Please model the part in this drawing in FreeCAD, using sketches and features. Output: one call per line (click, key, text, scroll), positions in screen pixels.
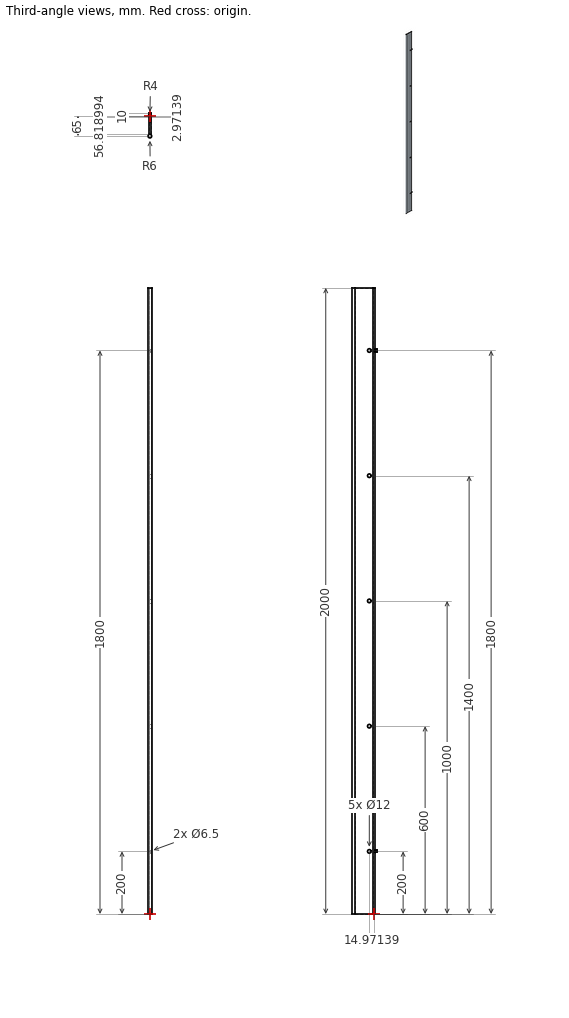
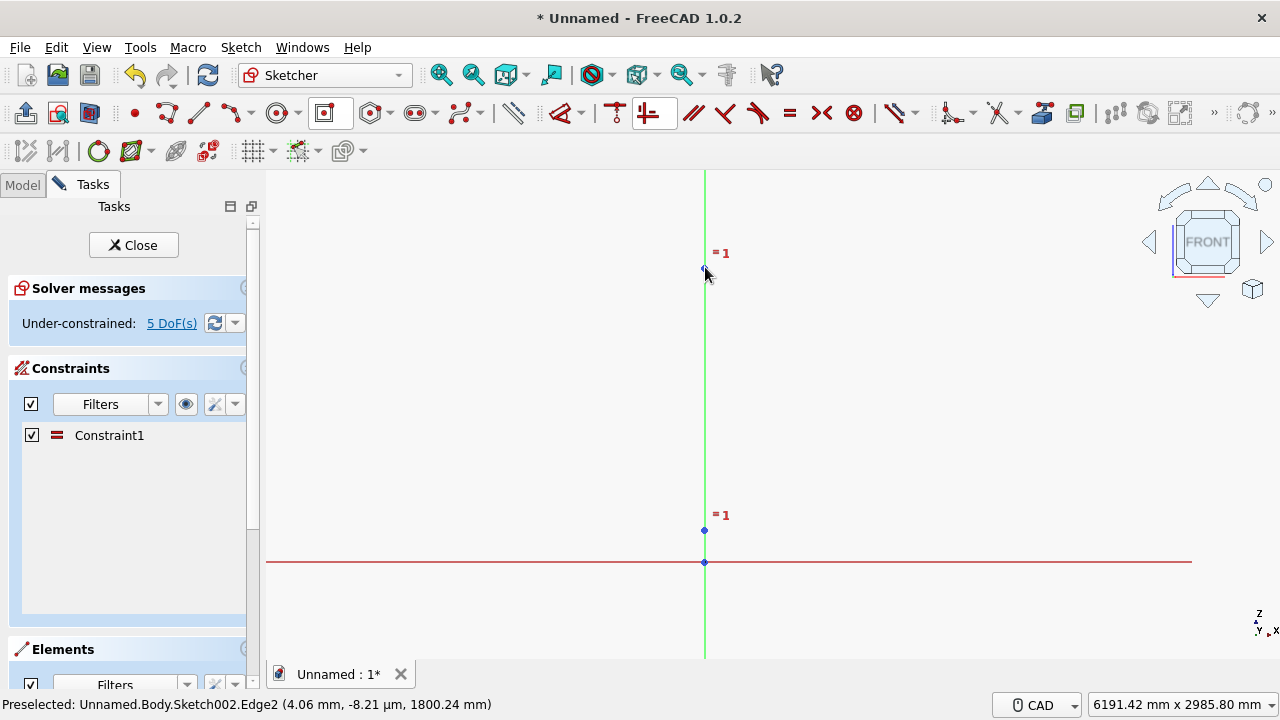
click(704, 531)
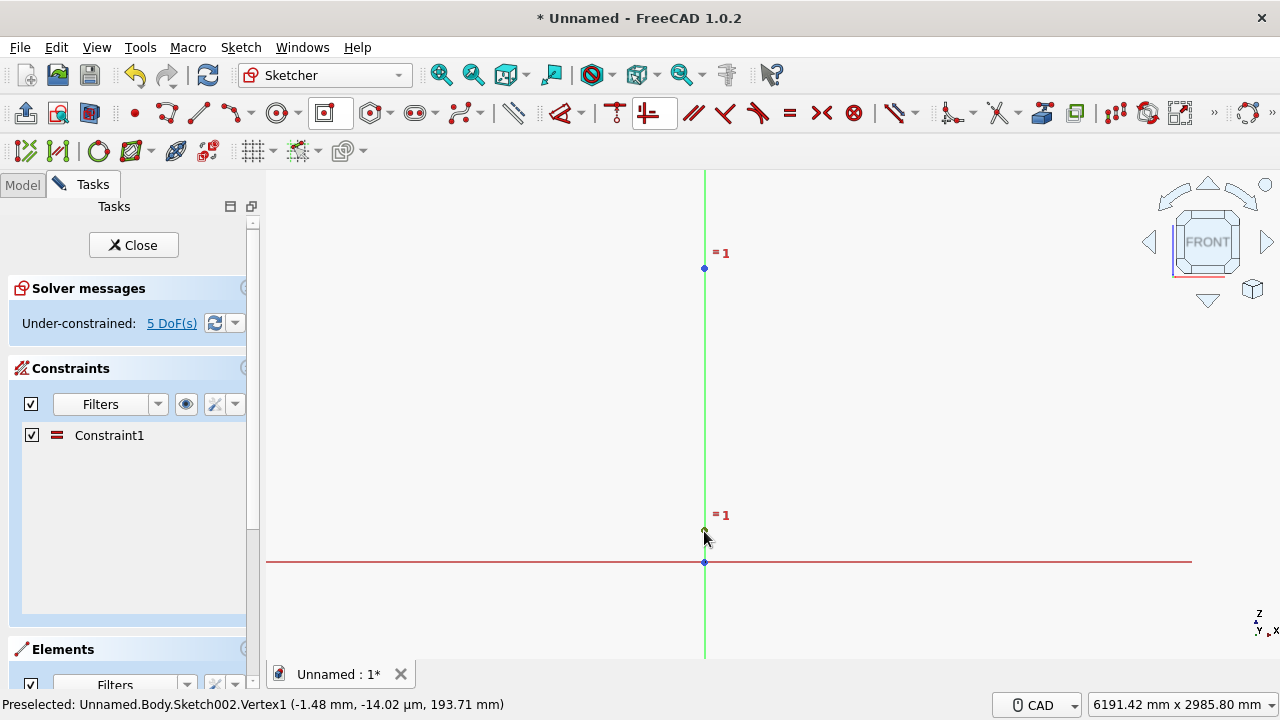
click(705, 600)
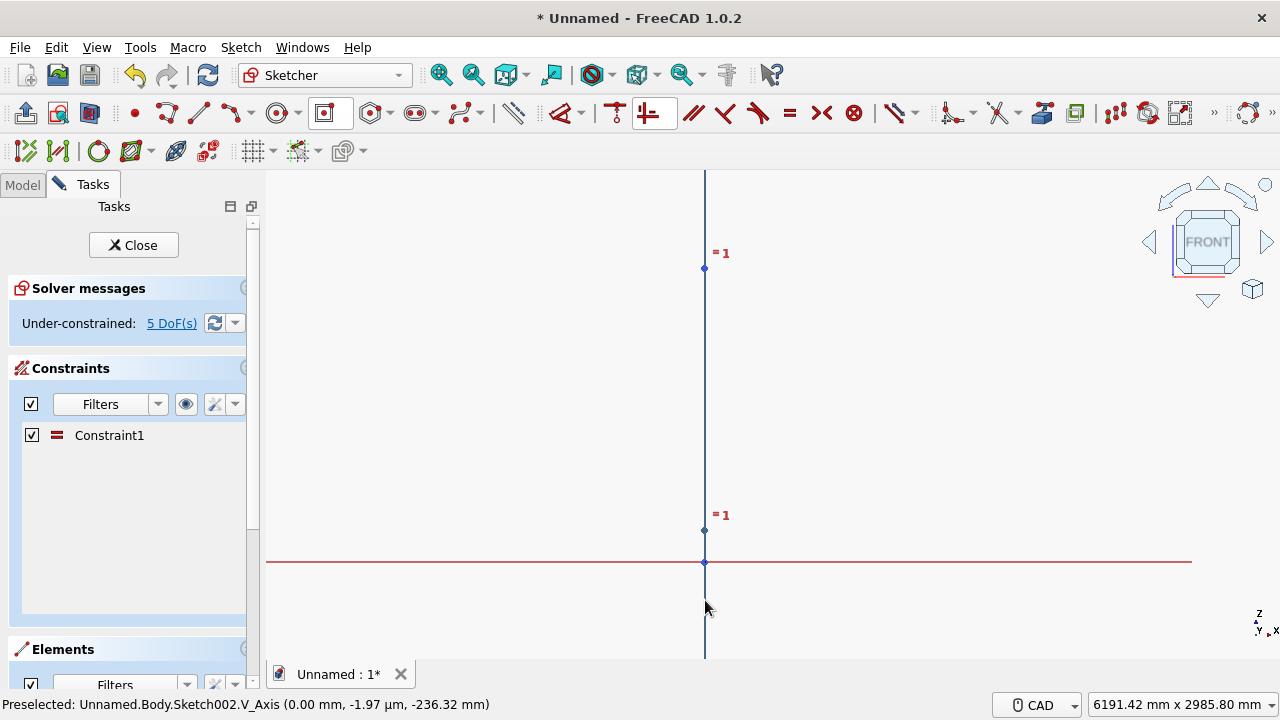
key(c)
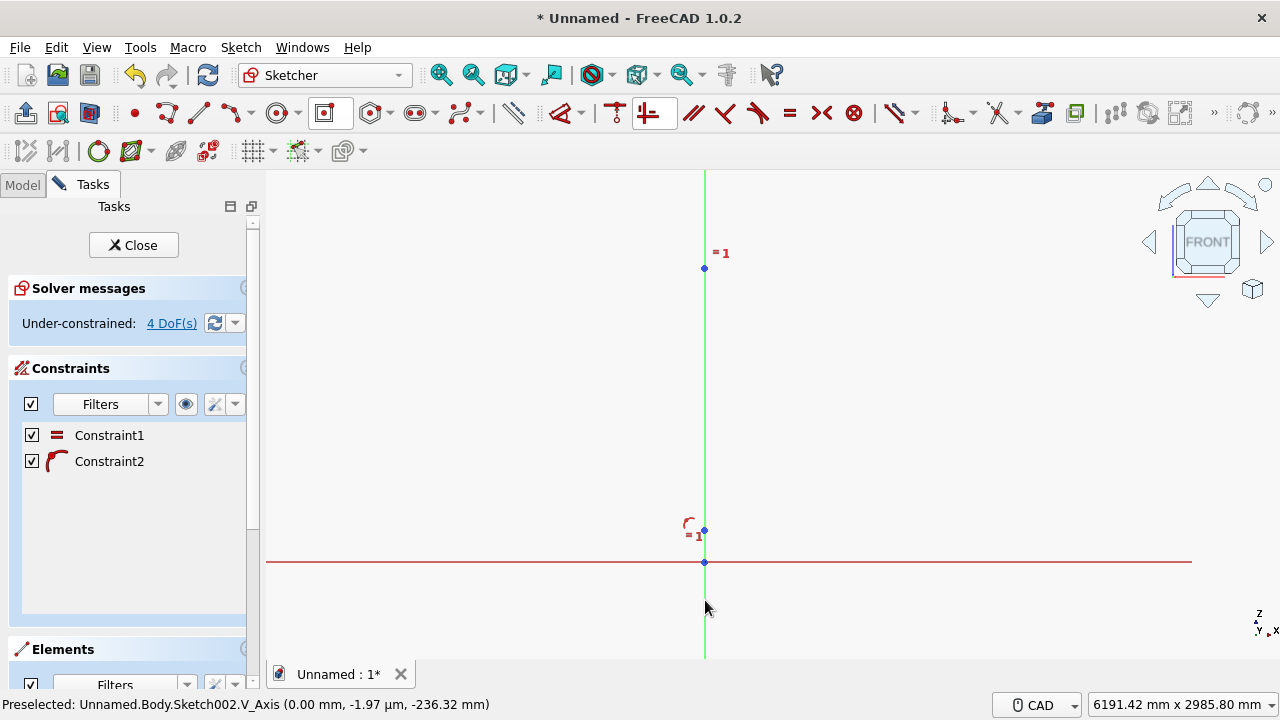
click(704, 269)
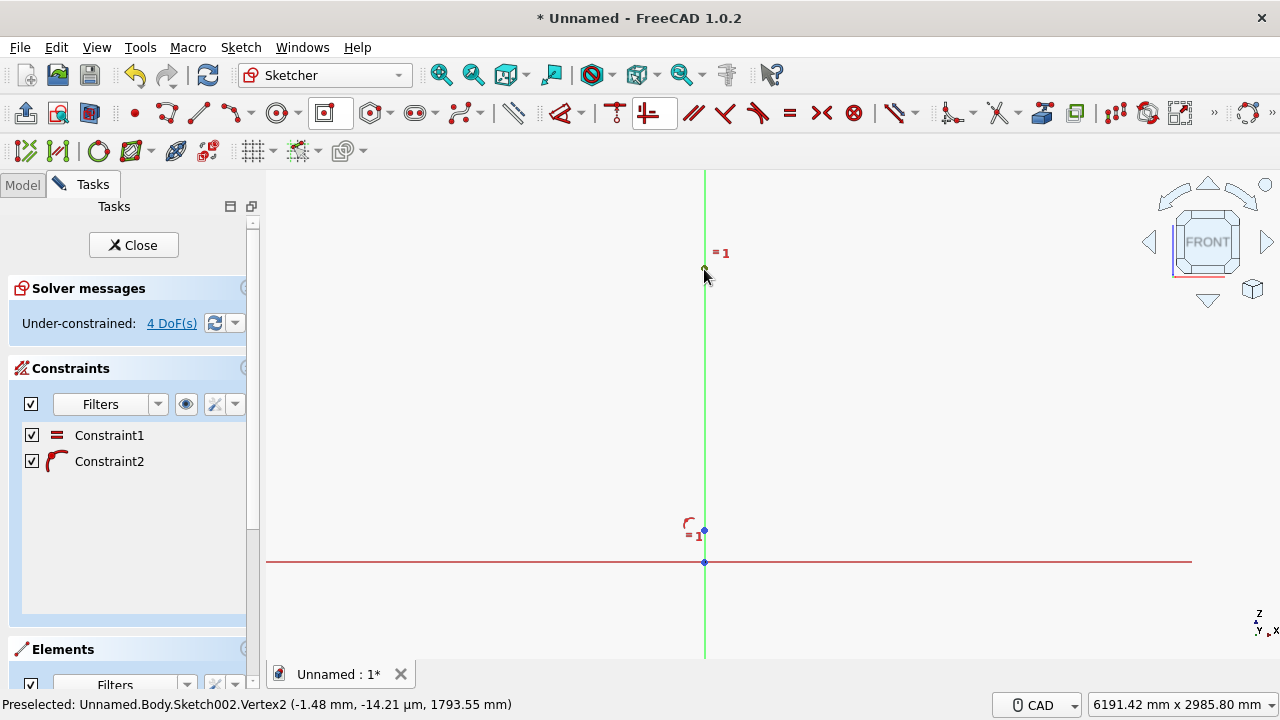
click(705, 600)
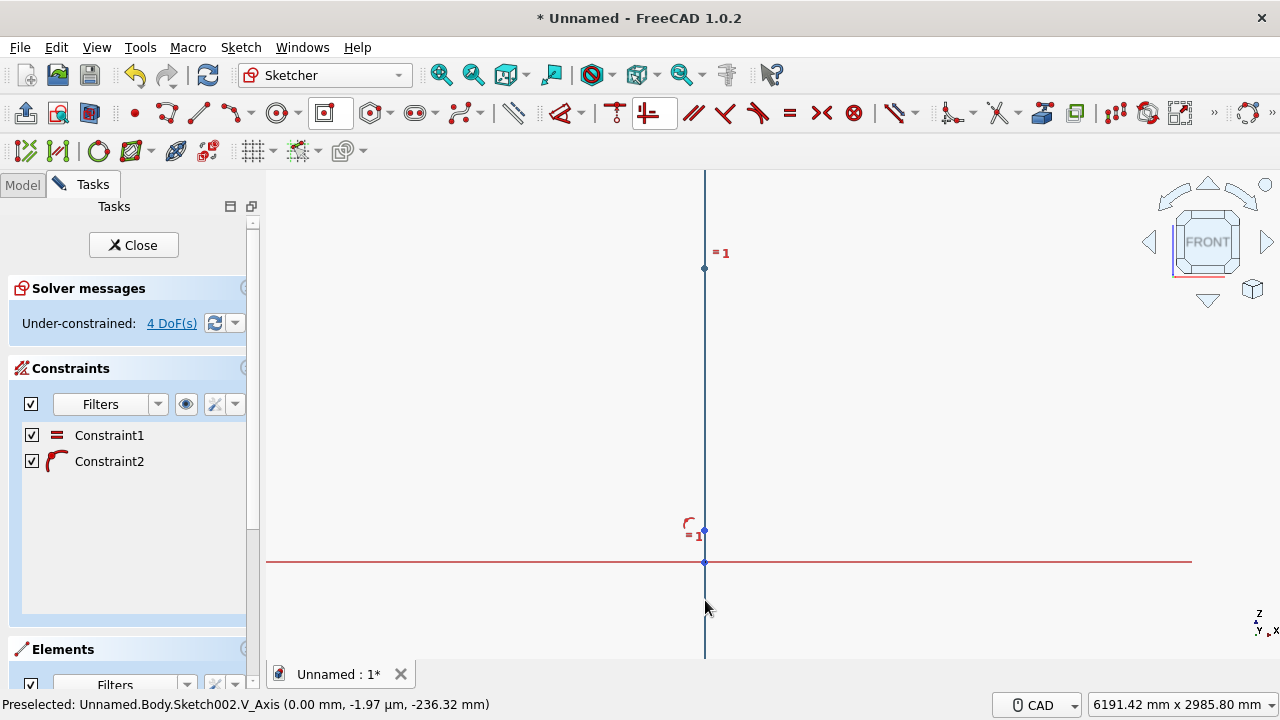
key(c)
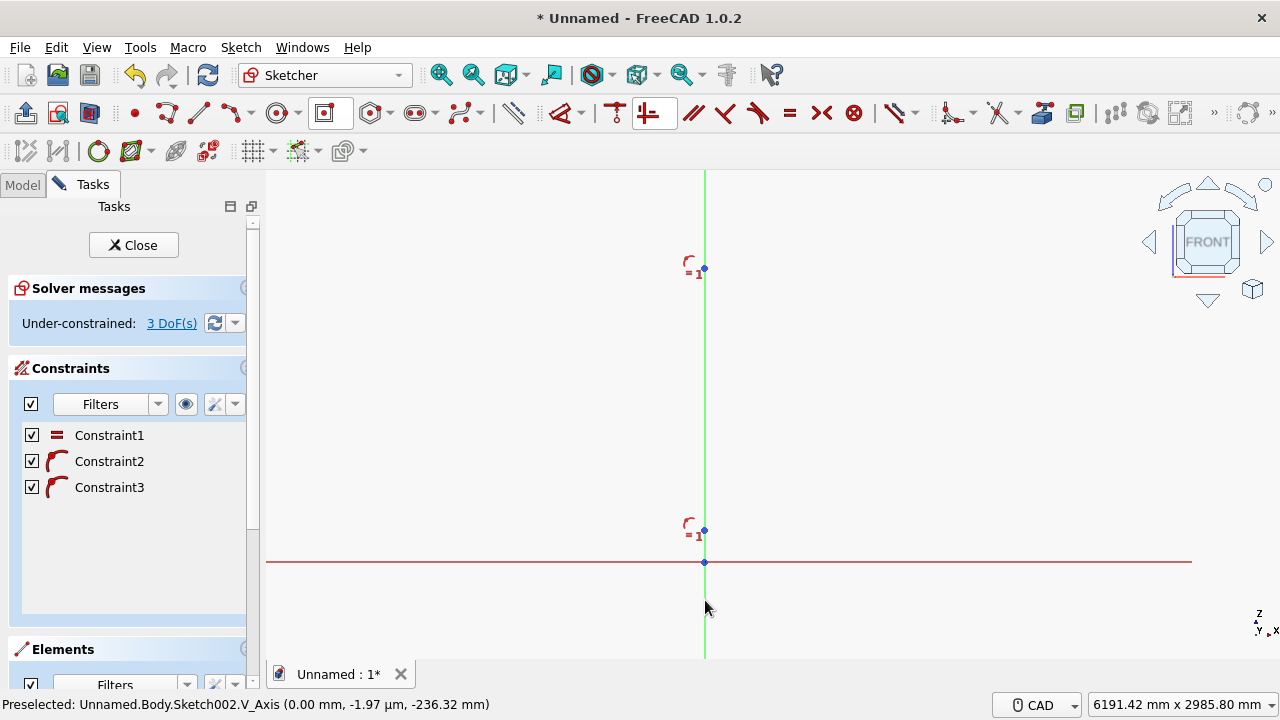
key(d)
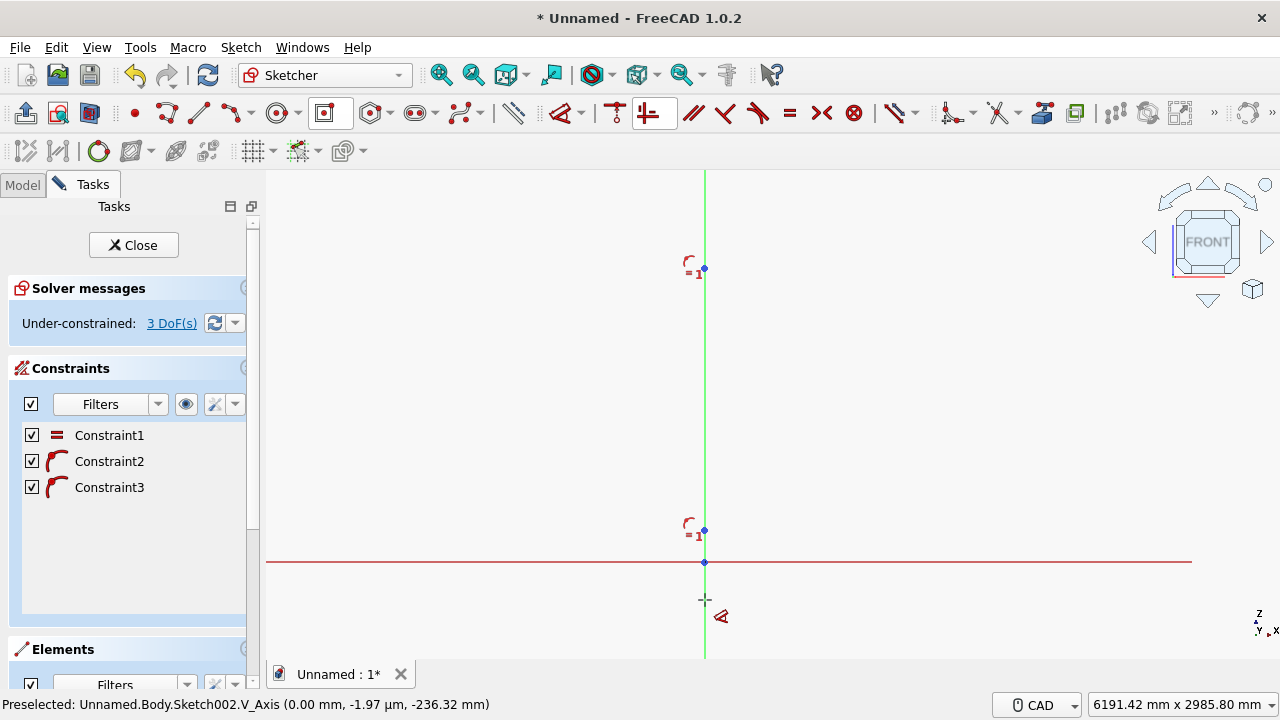
scroll(706, 530, up, 19)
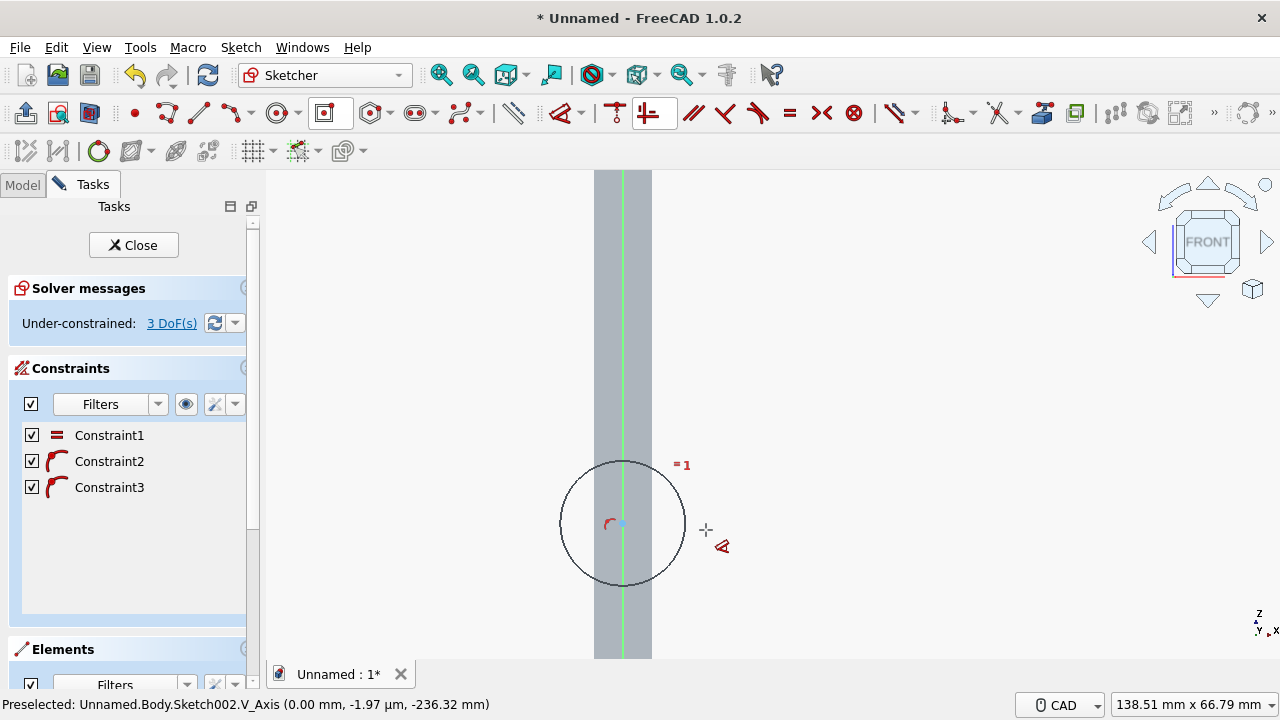
click(667, 479)
click(690, 456)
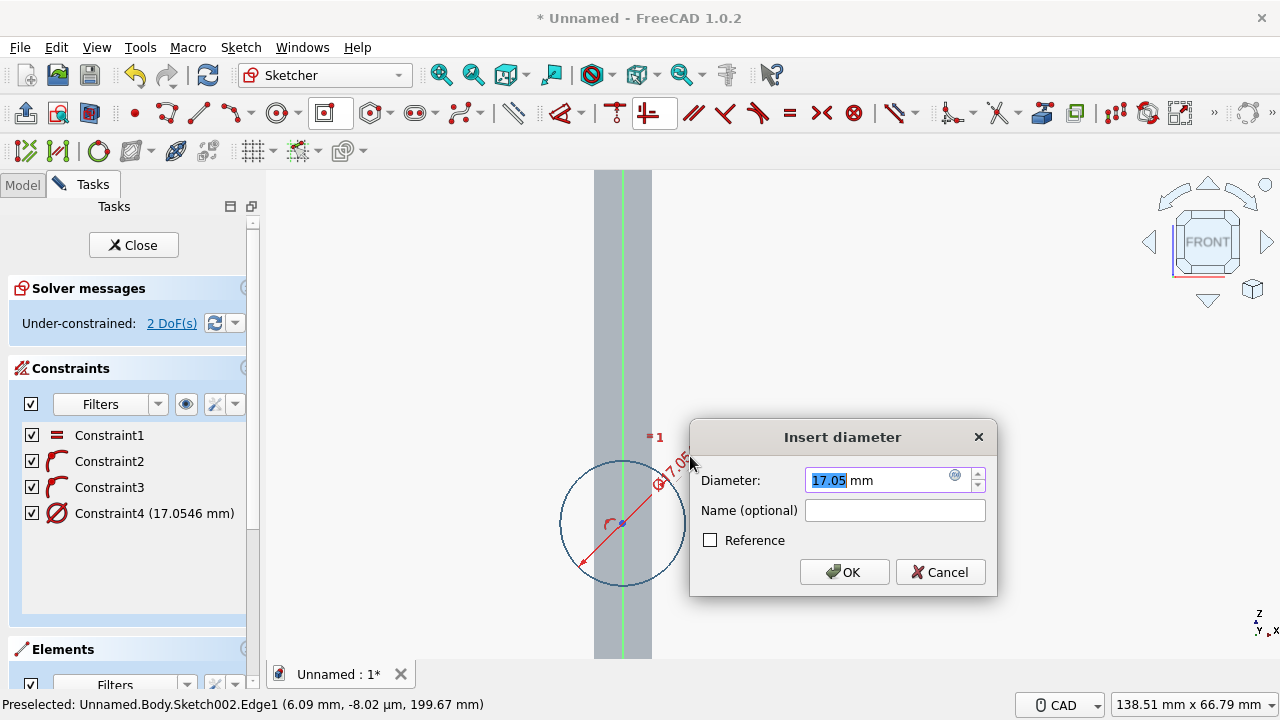
text(6.5)
key(Return)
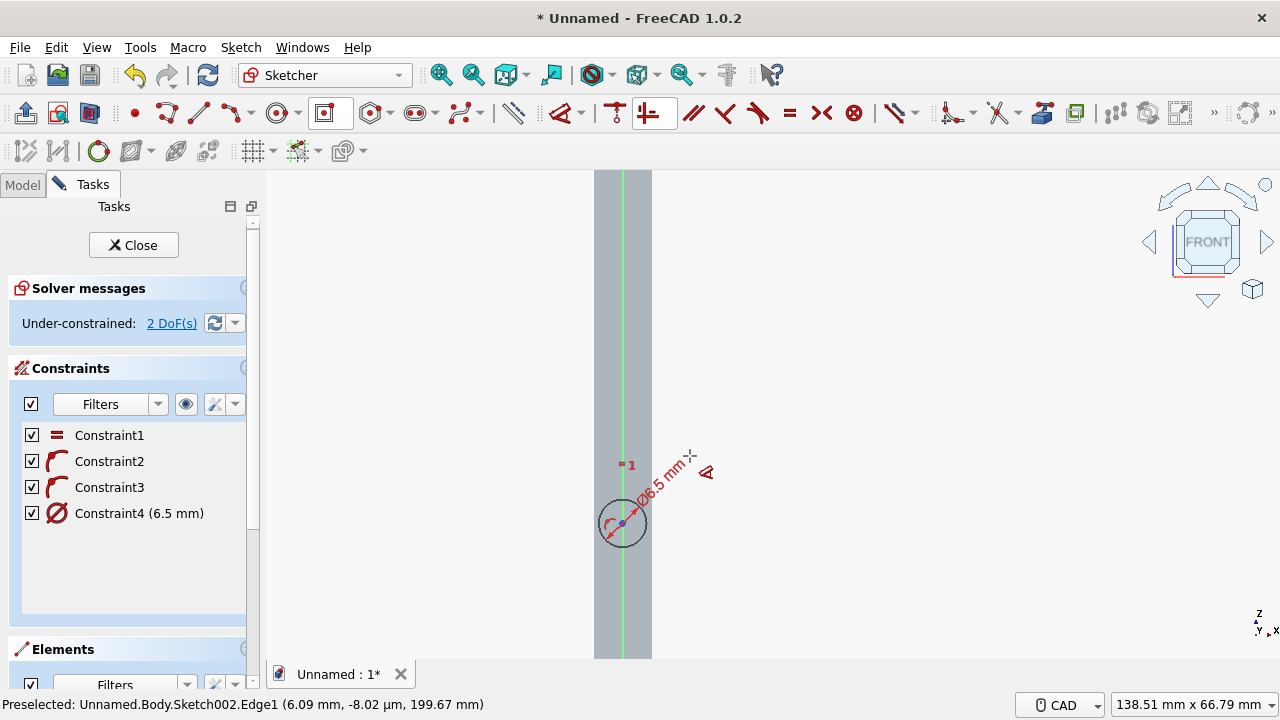
scroll(707, 557, down, 18)